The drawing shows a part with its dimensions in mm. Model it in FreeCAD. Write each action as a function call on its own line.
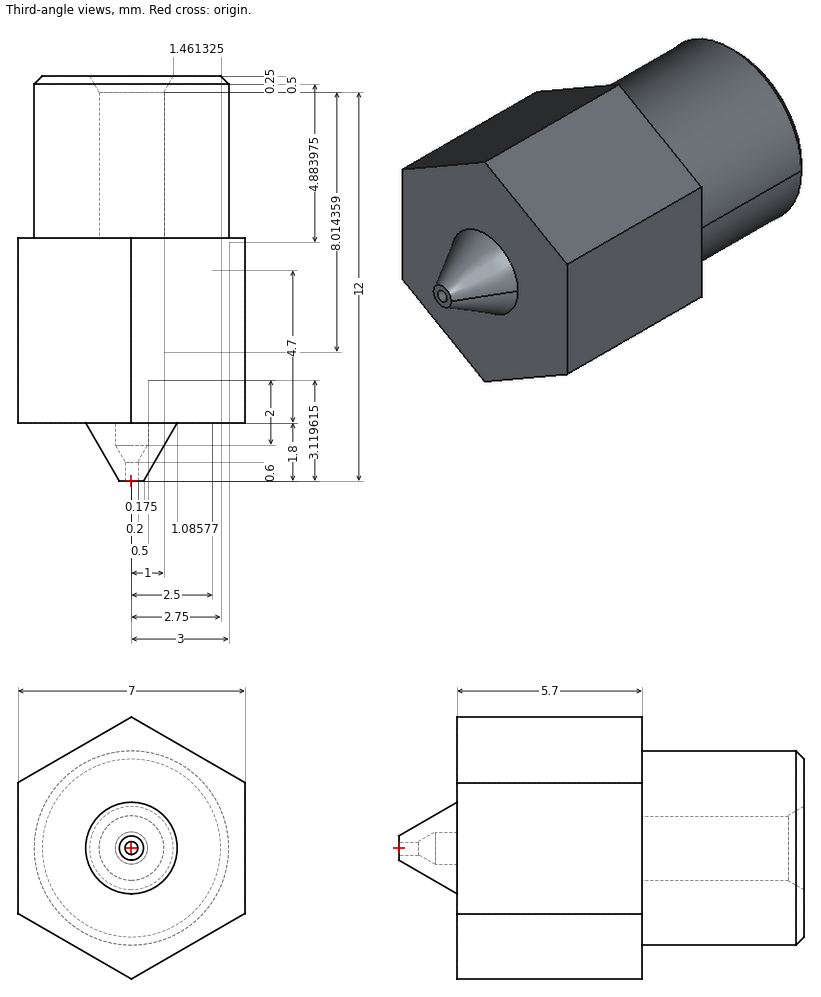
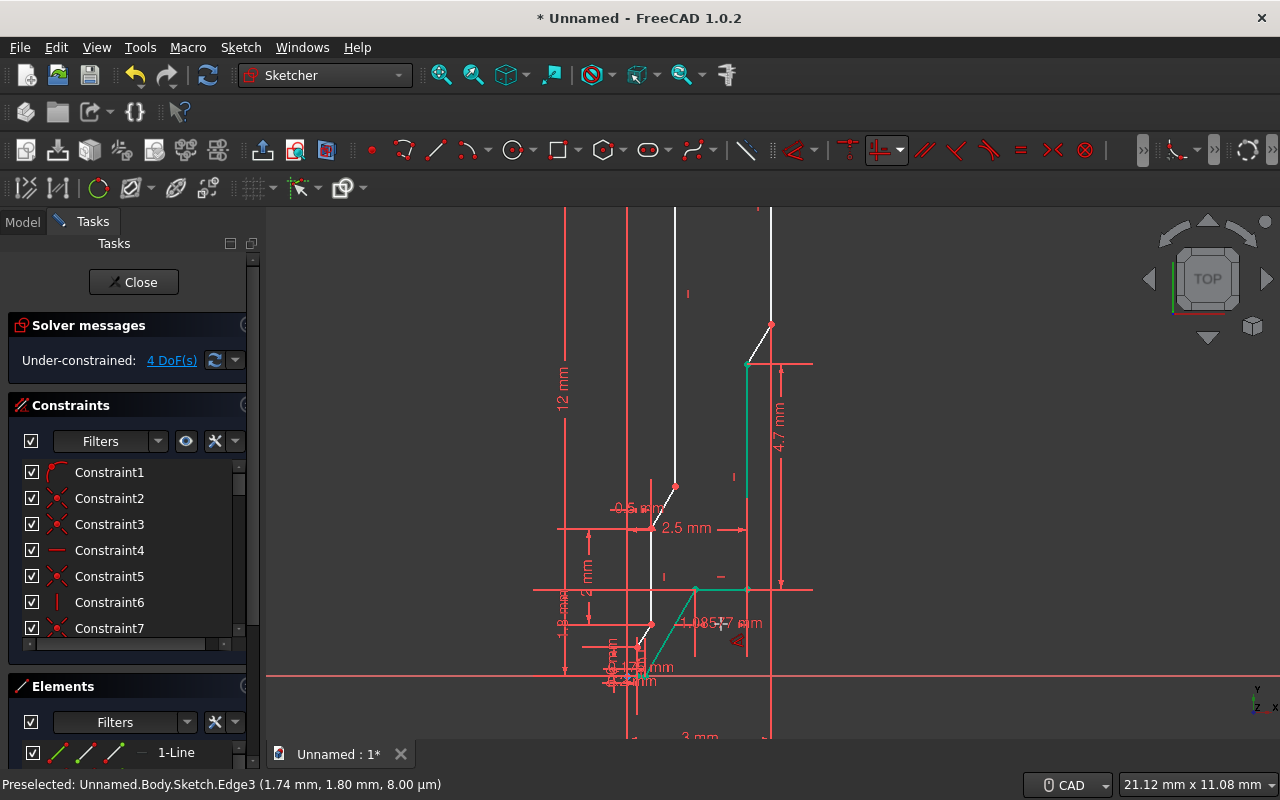
click(771, 253)
click(805, 280)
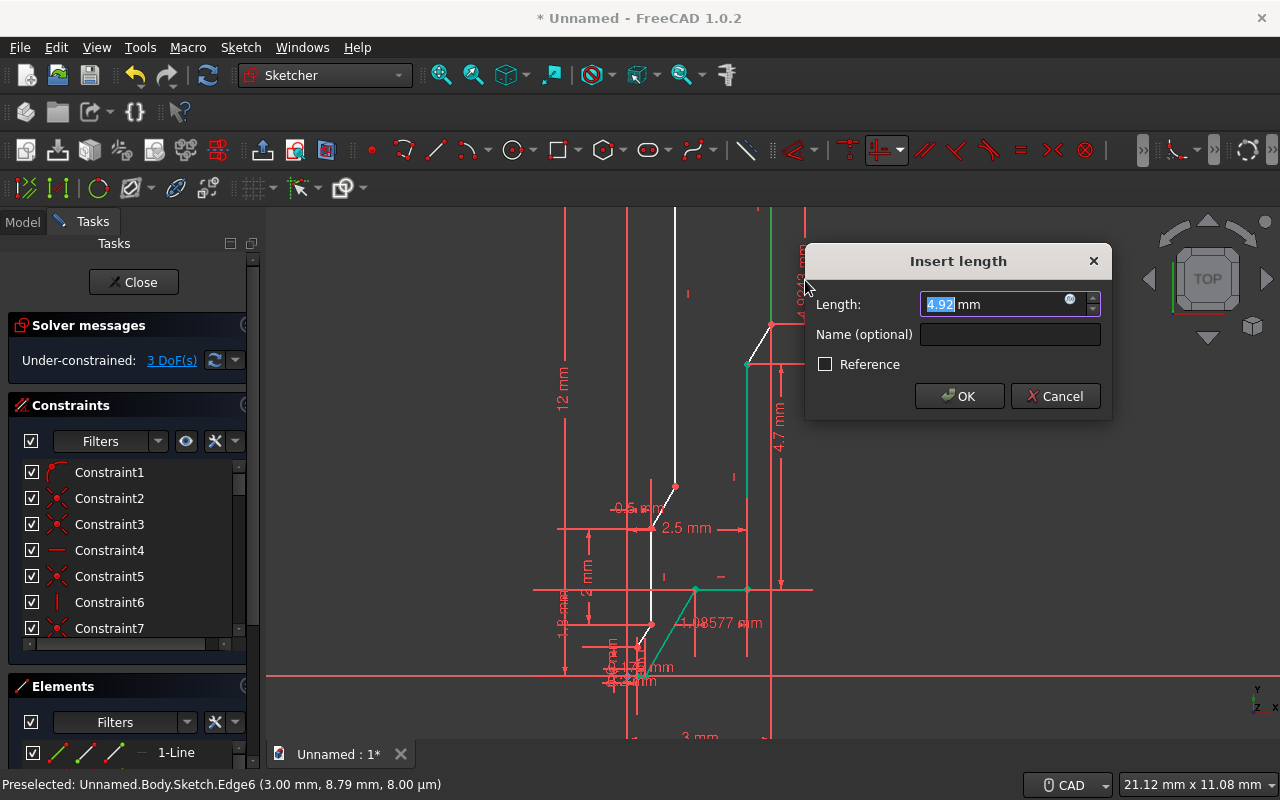
text(4.883975)
key(Return)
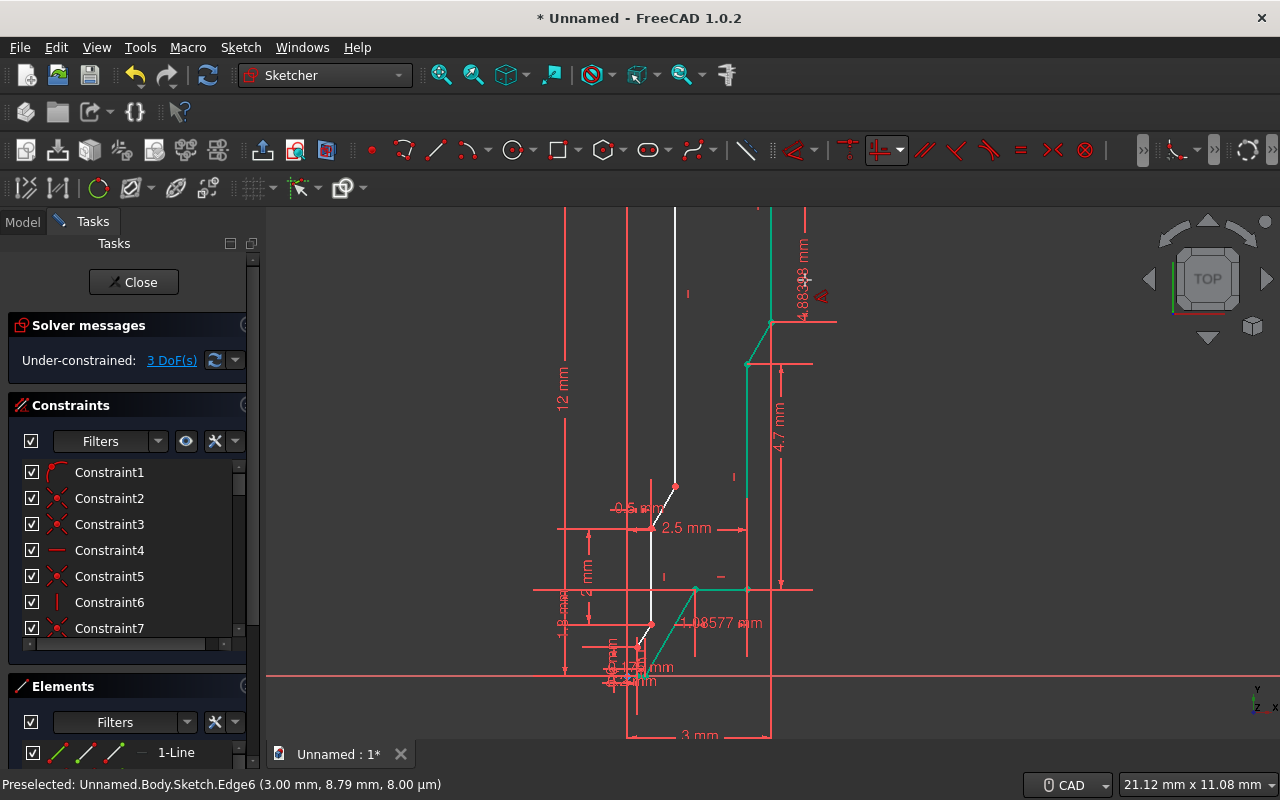
scroll(711, 591, down, 3)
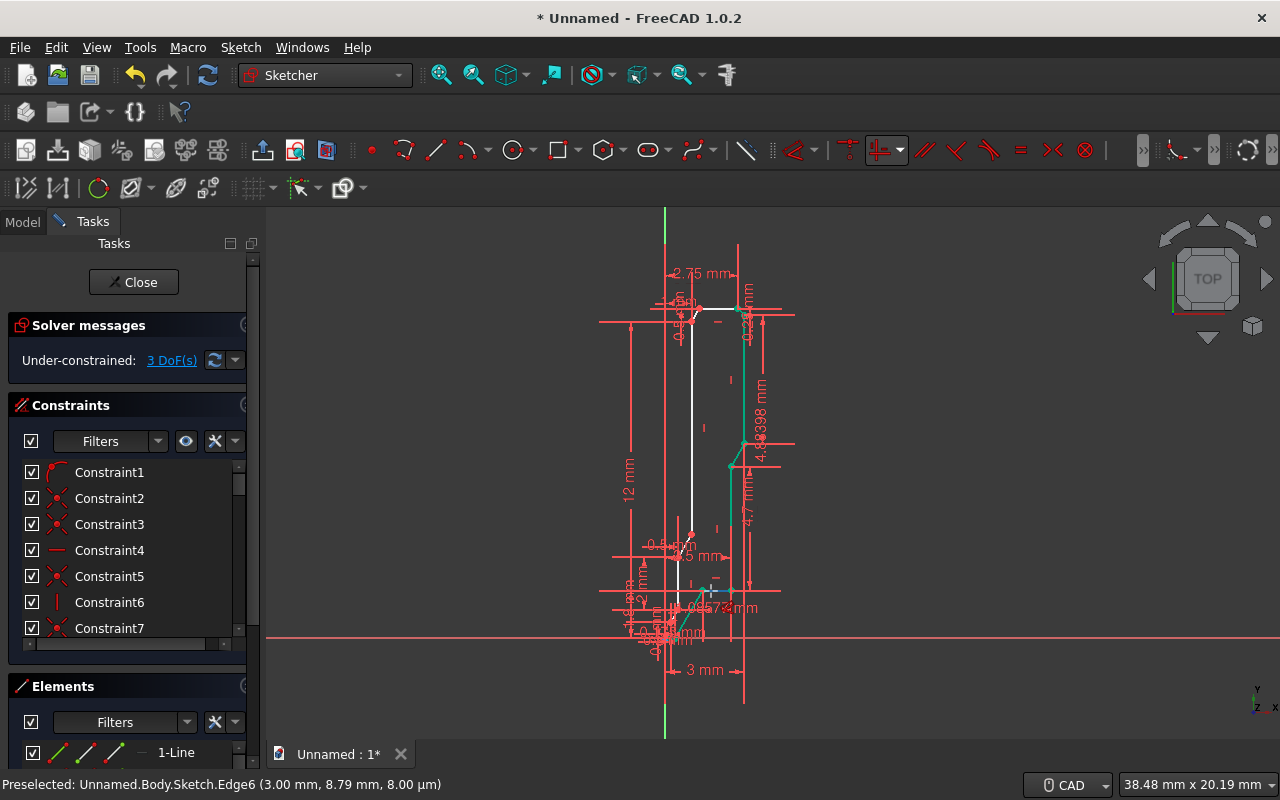
click(726, 309)
click(718, 343)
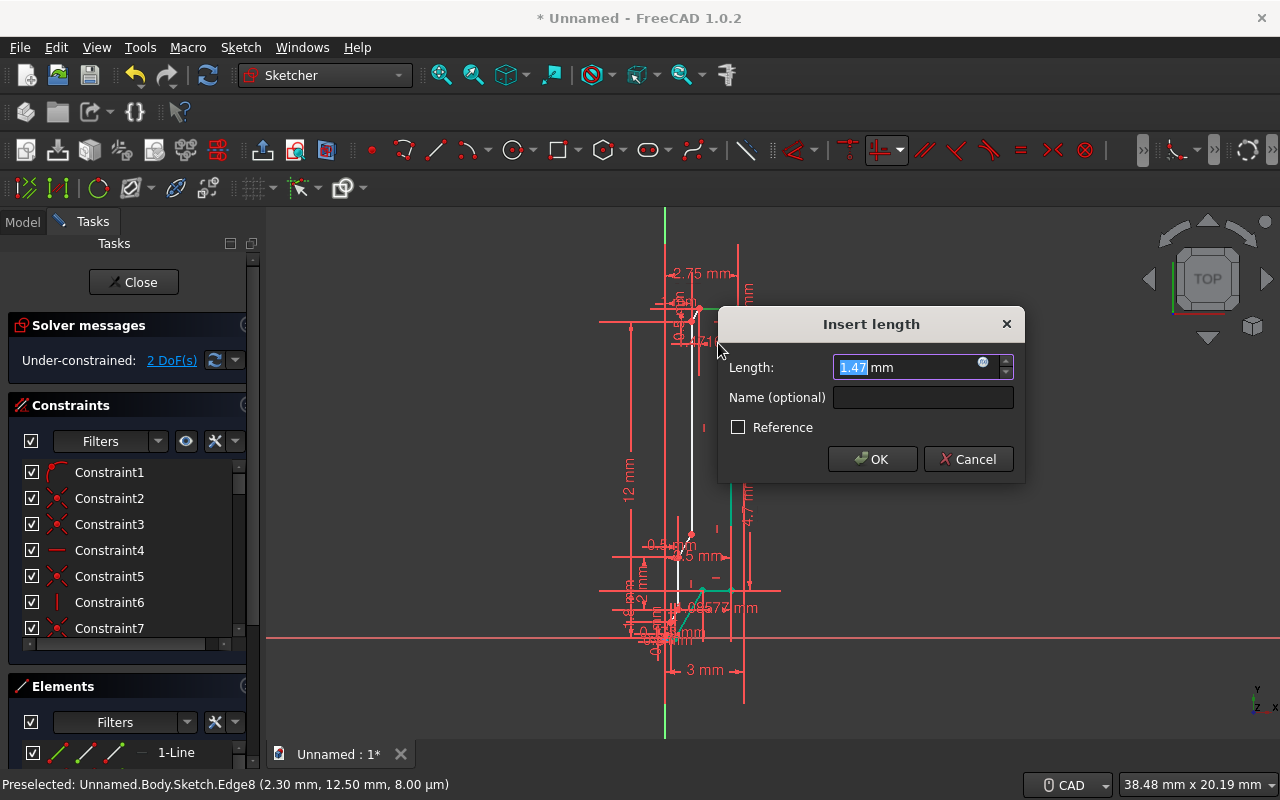
text(1.461325)
key(Return)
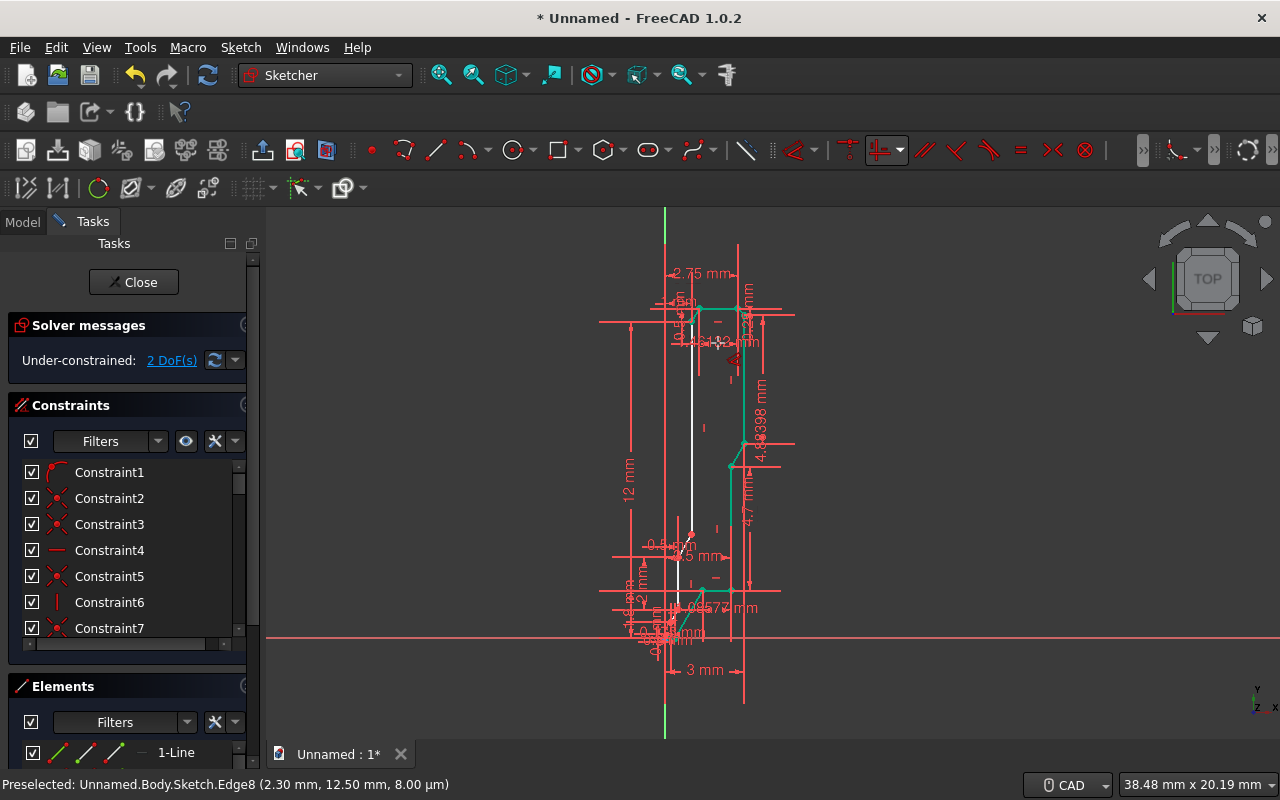
click(692, 386)
click(726, 379)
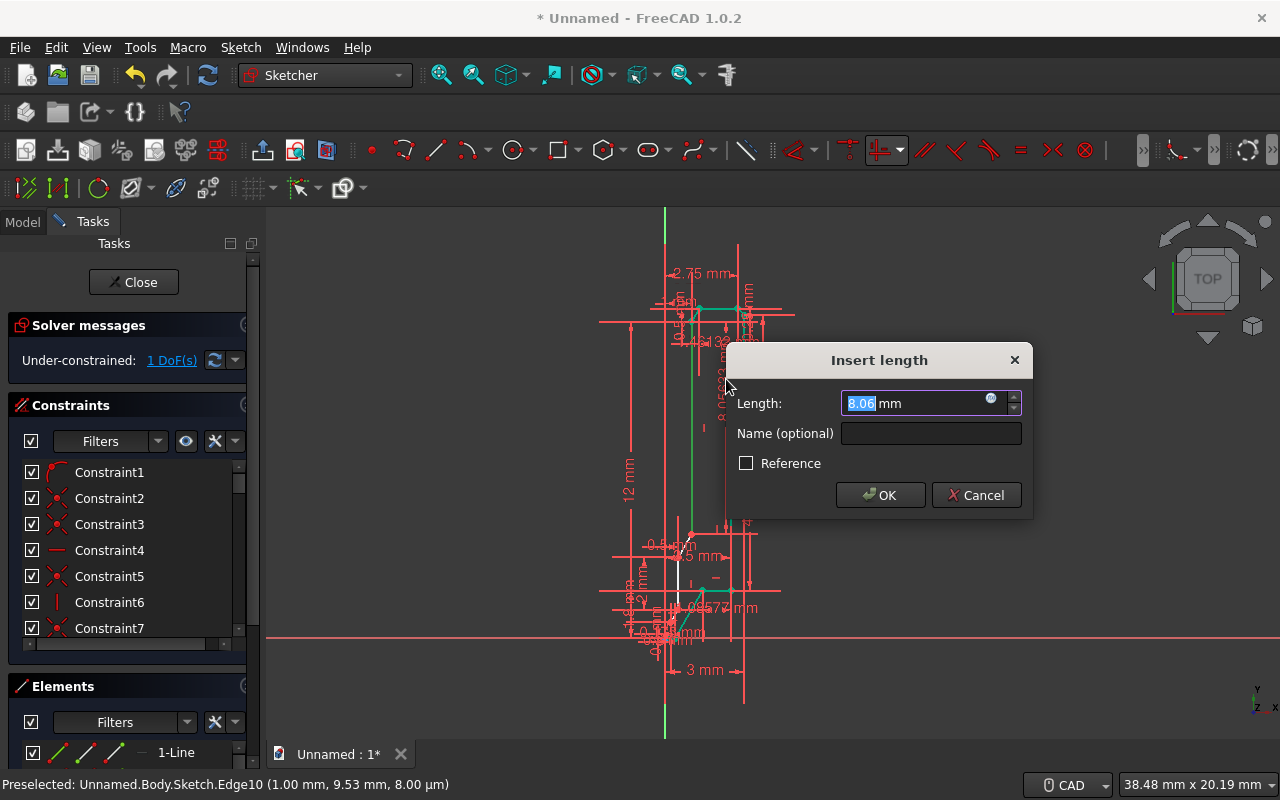
text(8.014359)
key(Return)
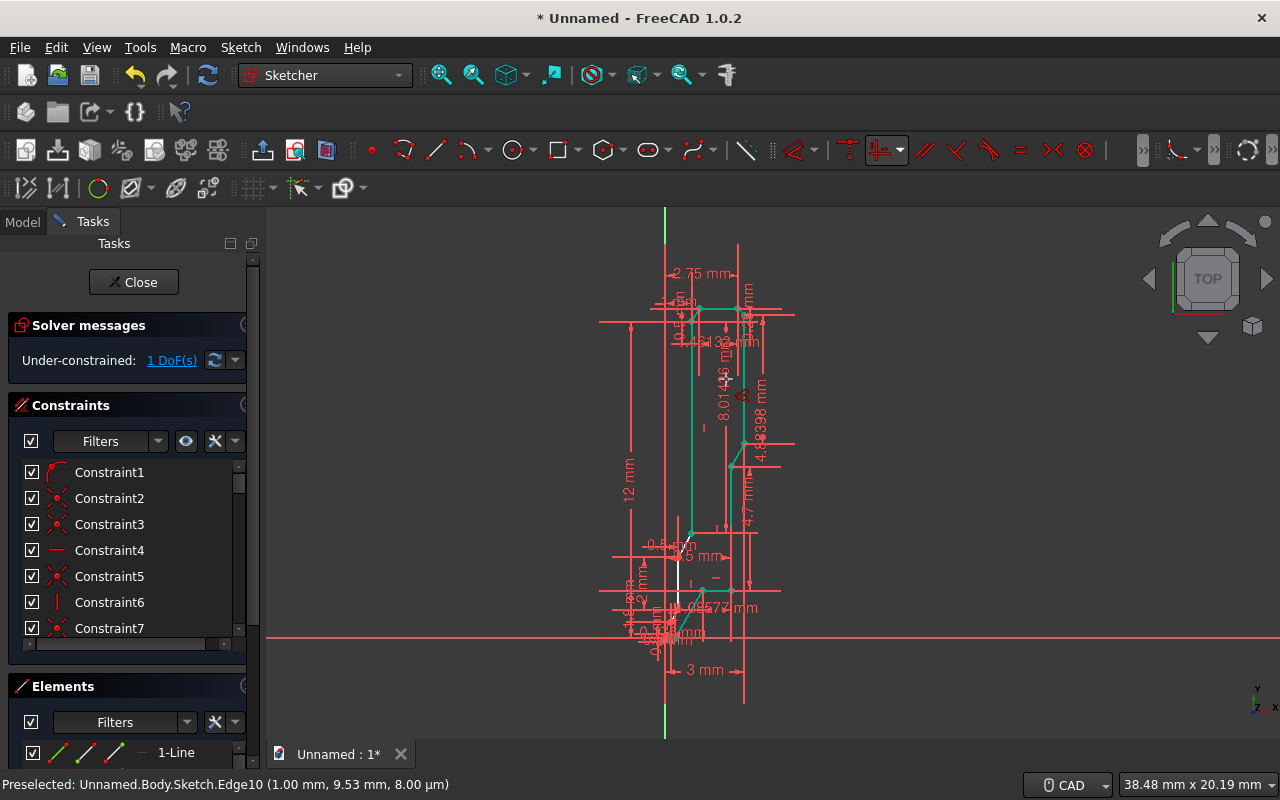
click(679, 557)
click(761, 579)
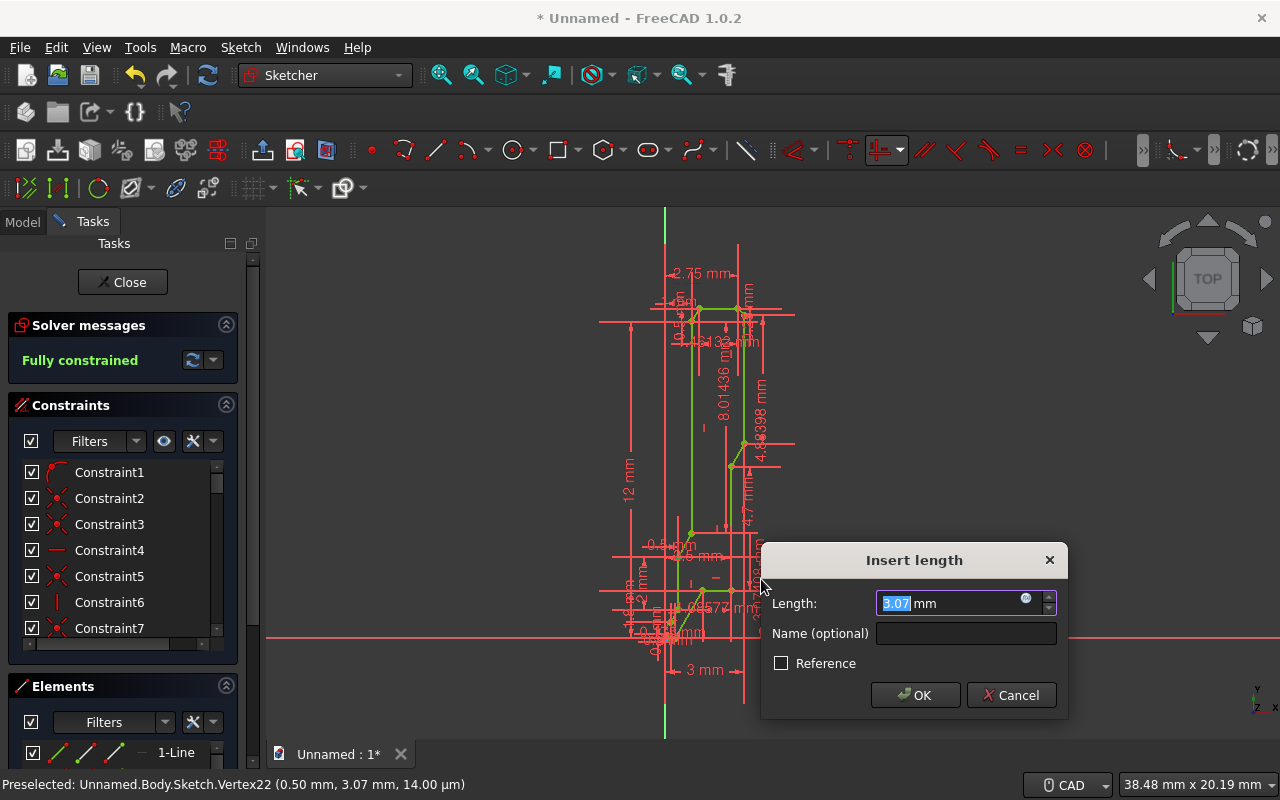
text(3.119615)
key(Return)
key(Escape)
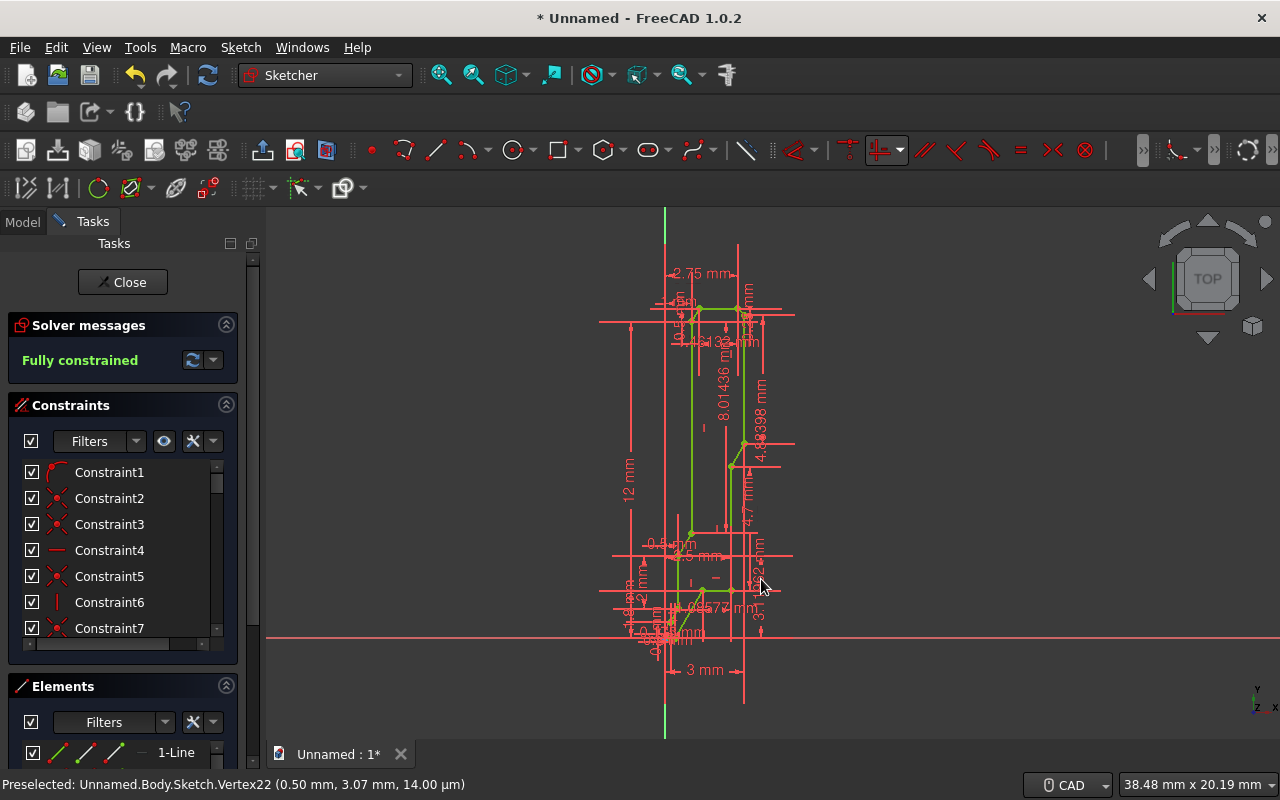
click(123, 282)